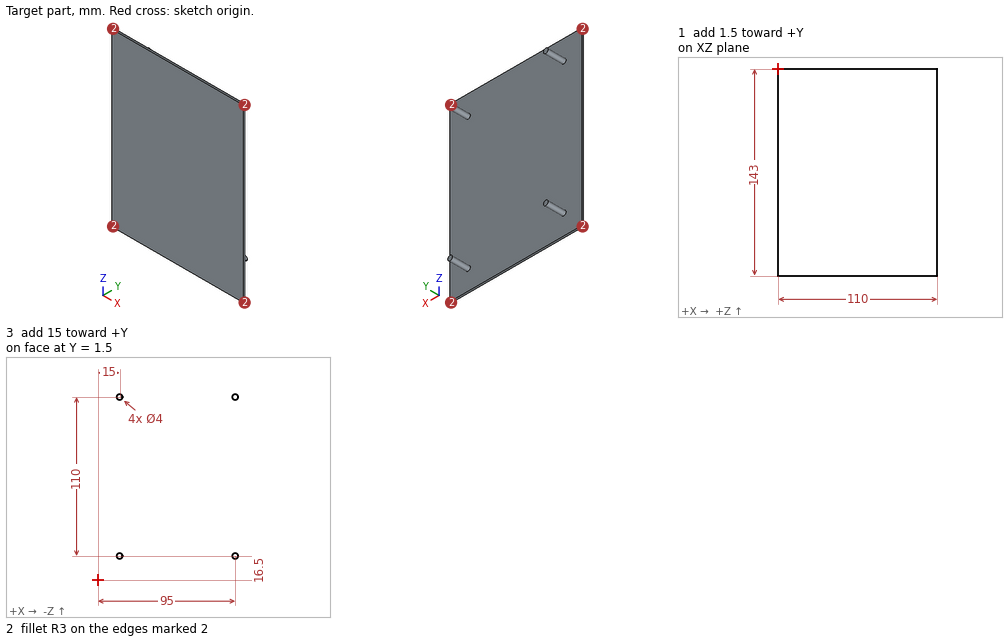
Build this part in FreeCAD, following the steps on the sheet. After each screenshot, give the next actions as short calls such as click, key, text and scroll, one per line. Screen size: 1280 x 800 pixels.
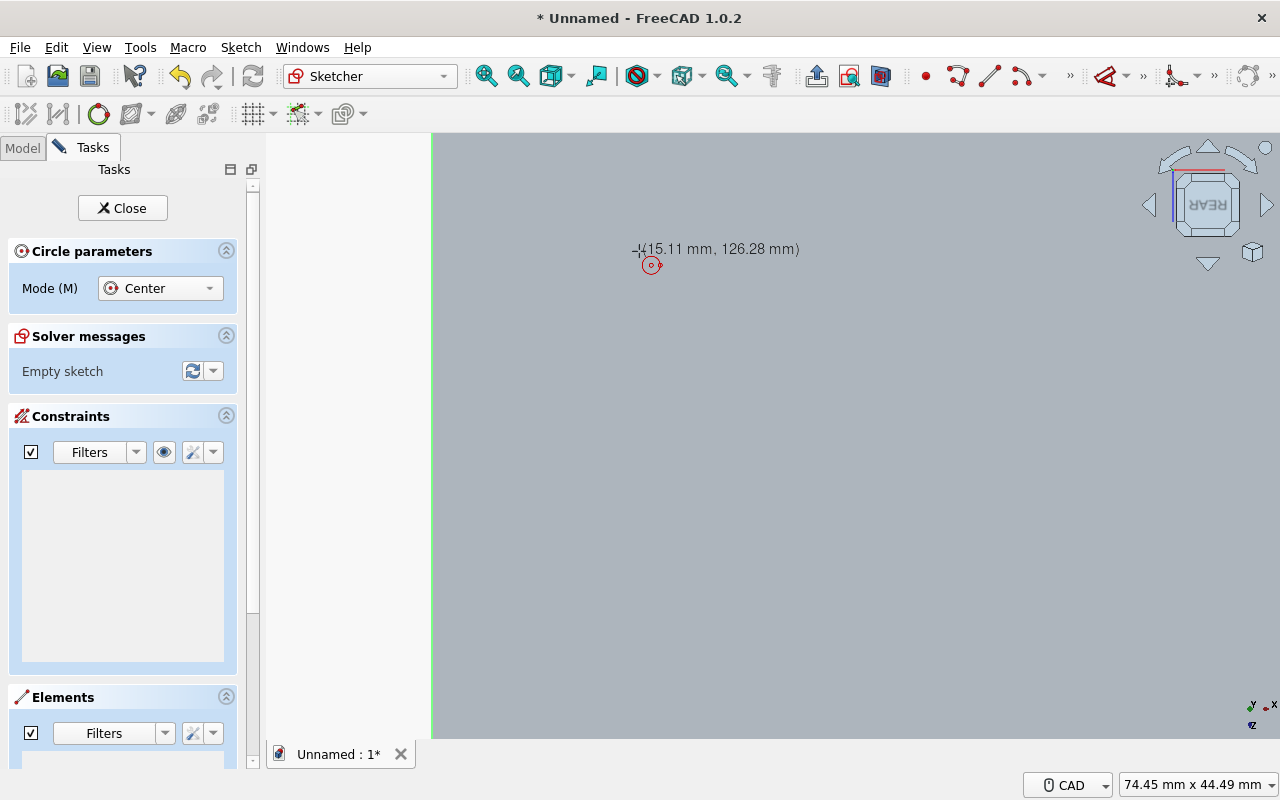
scroll(606, 268, down, 8)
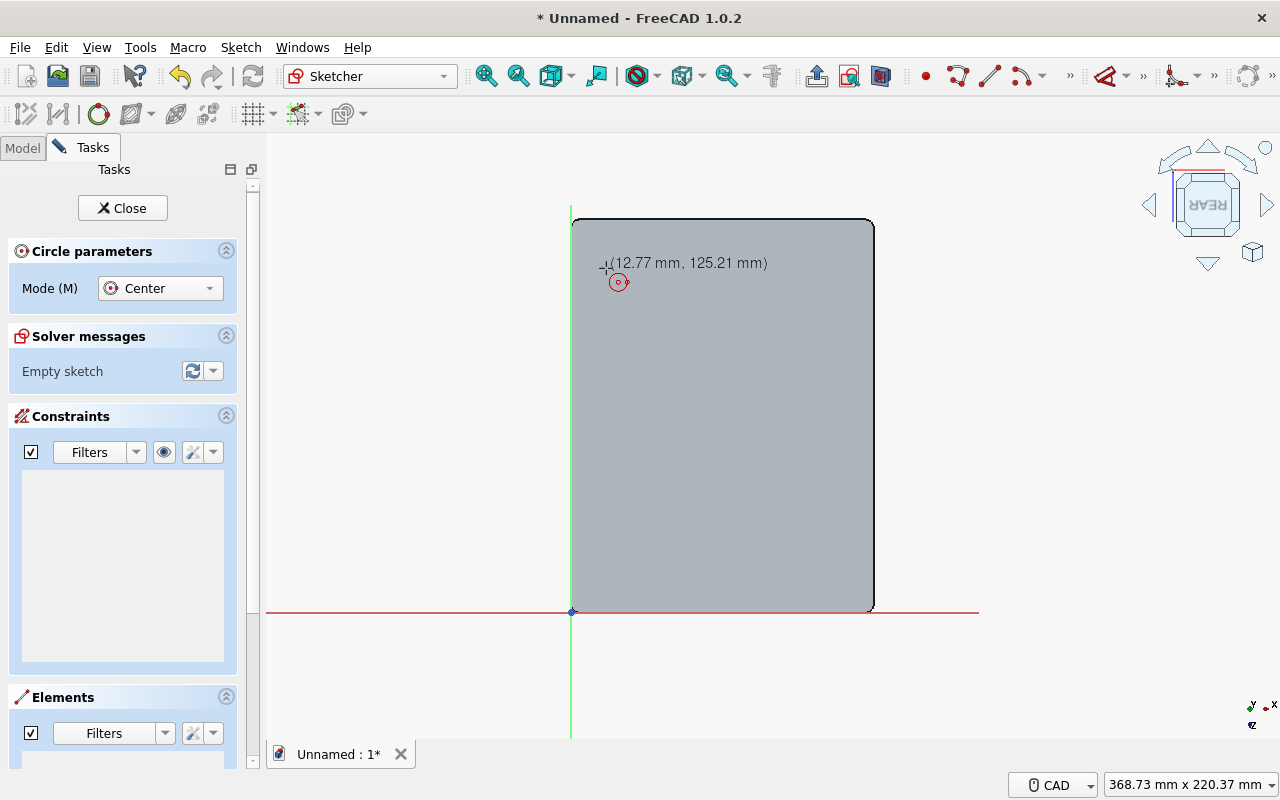
click(612, 265)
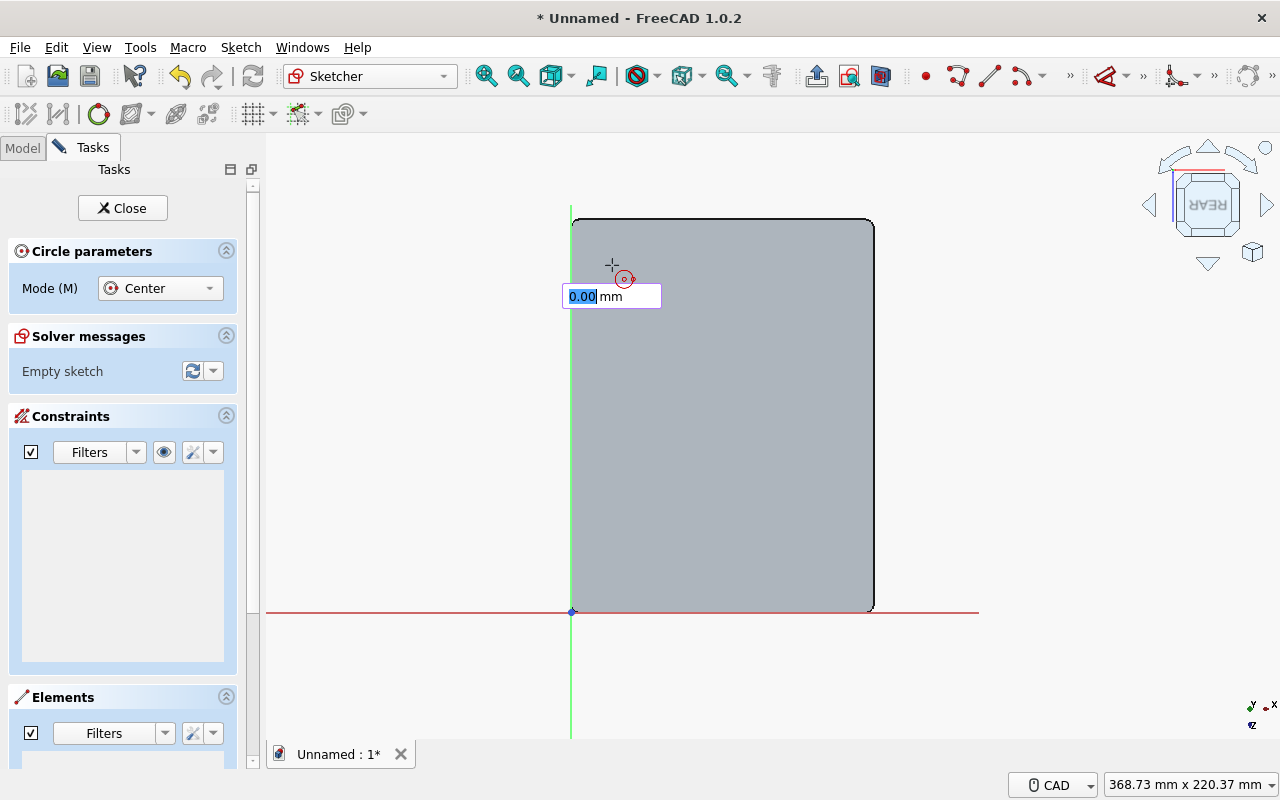
scroll(616, 261, up, 6)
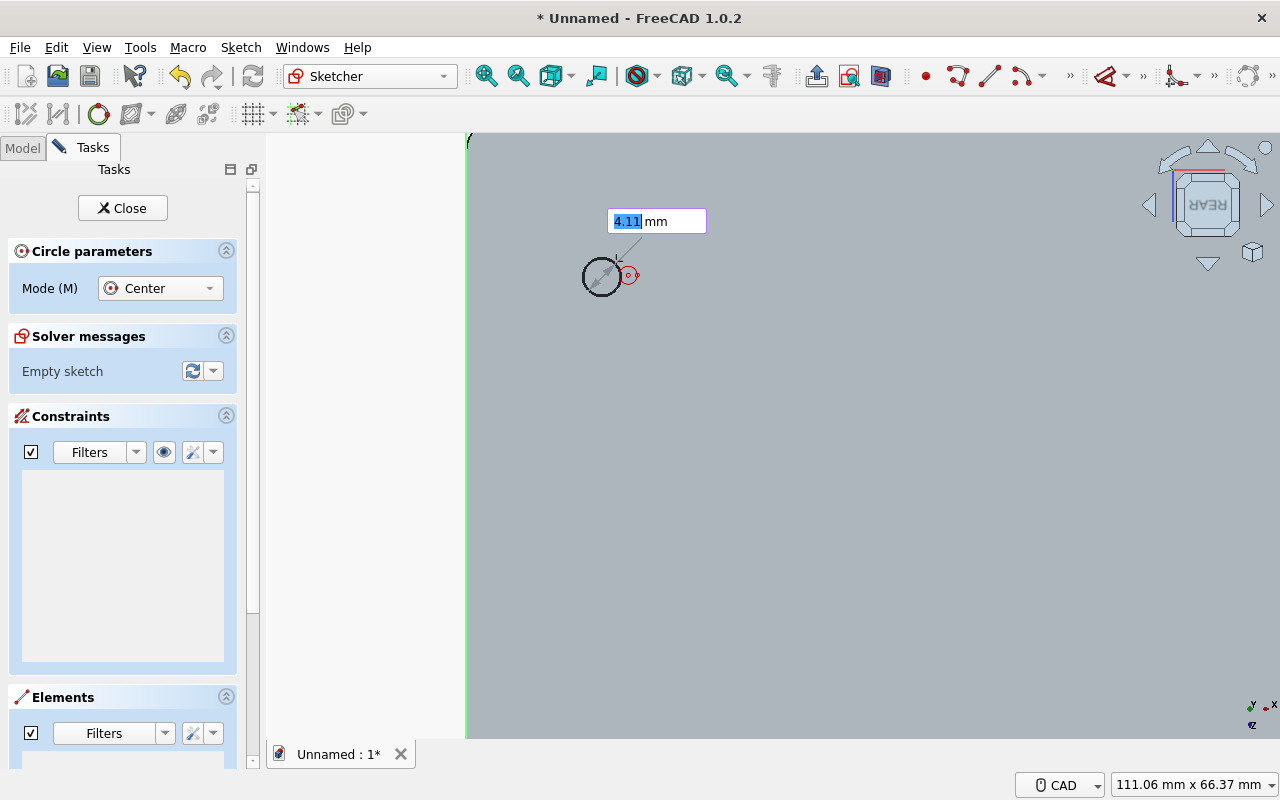
click(616, 260)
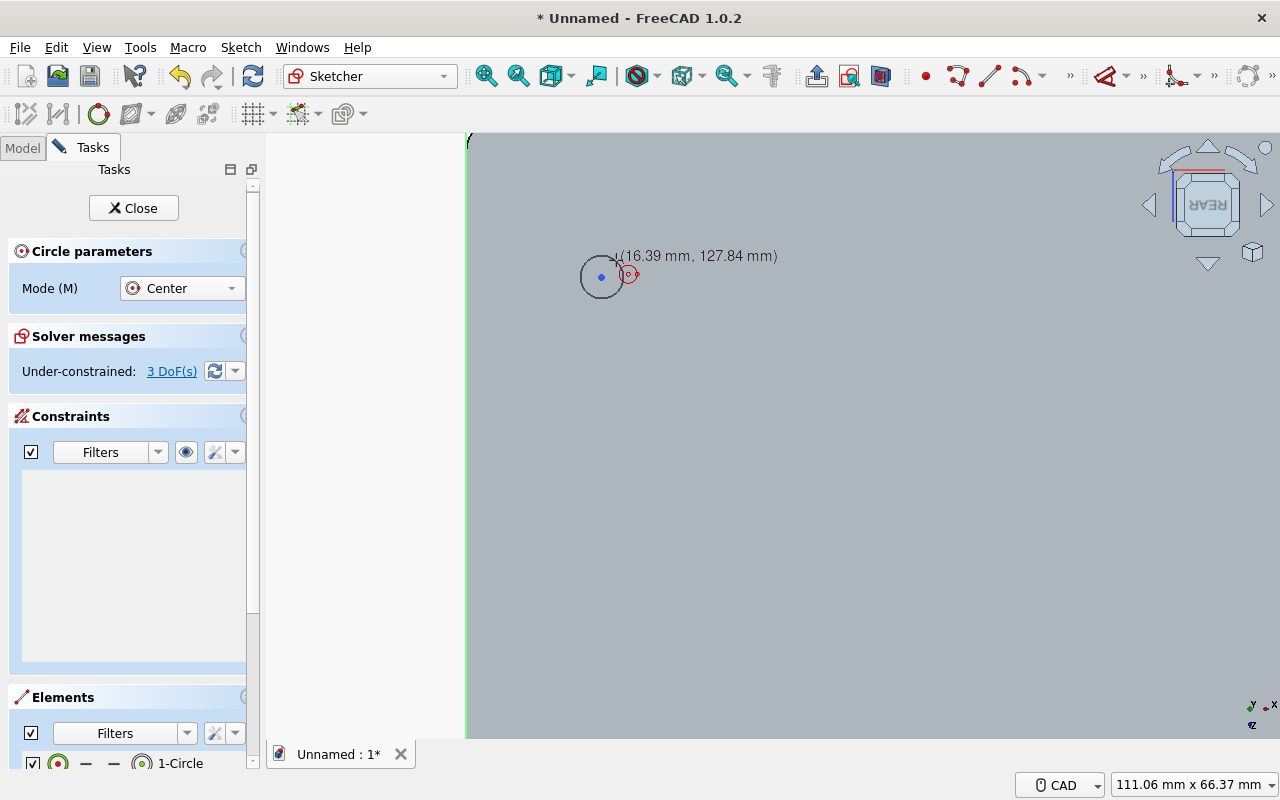
scroll(616, 261, down, 6)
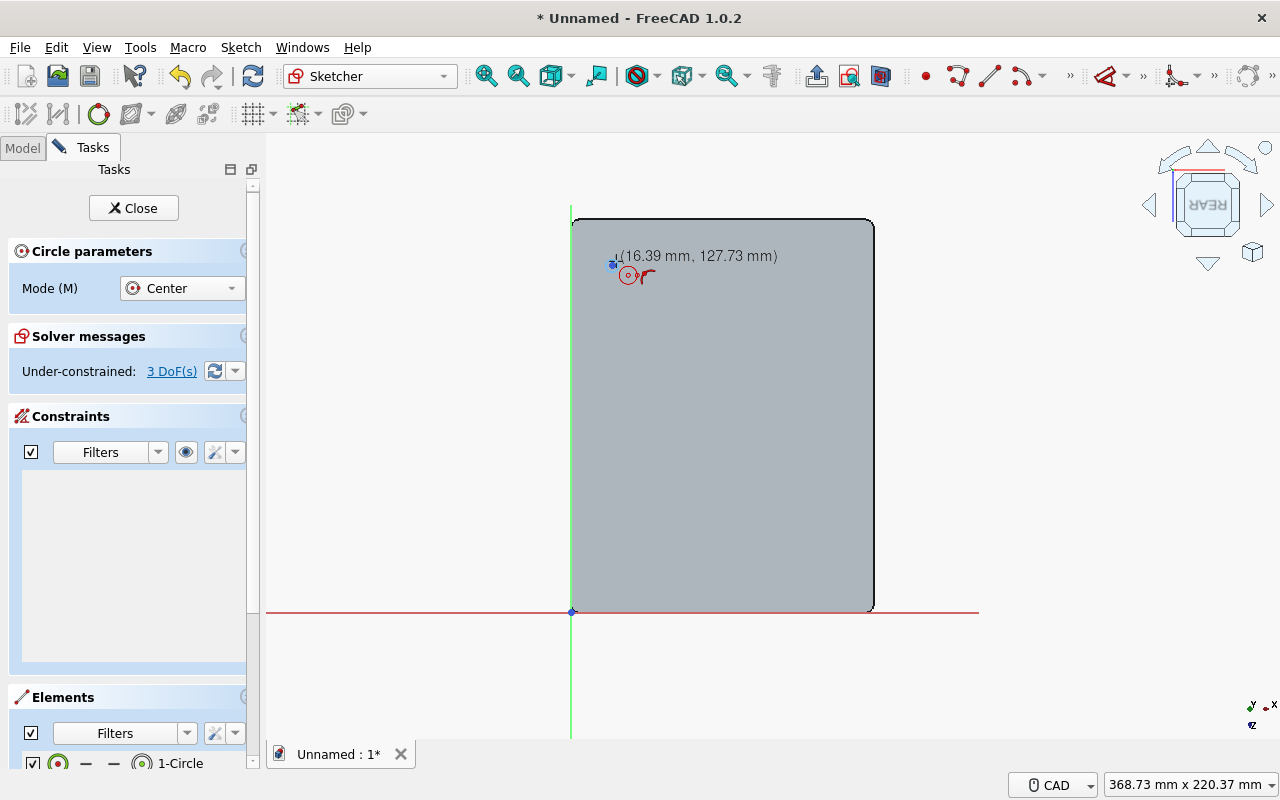
scroll(832, 567, up, 8)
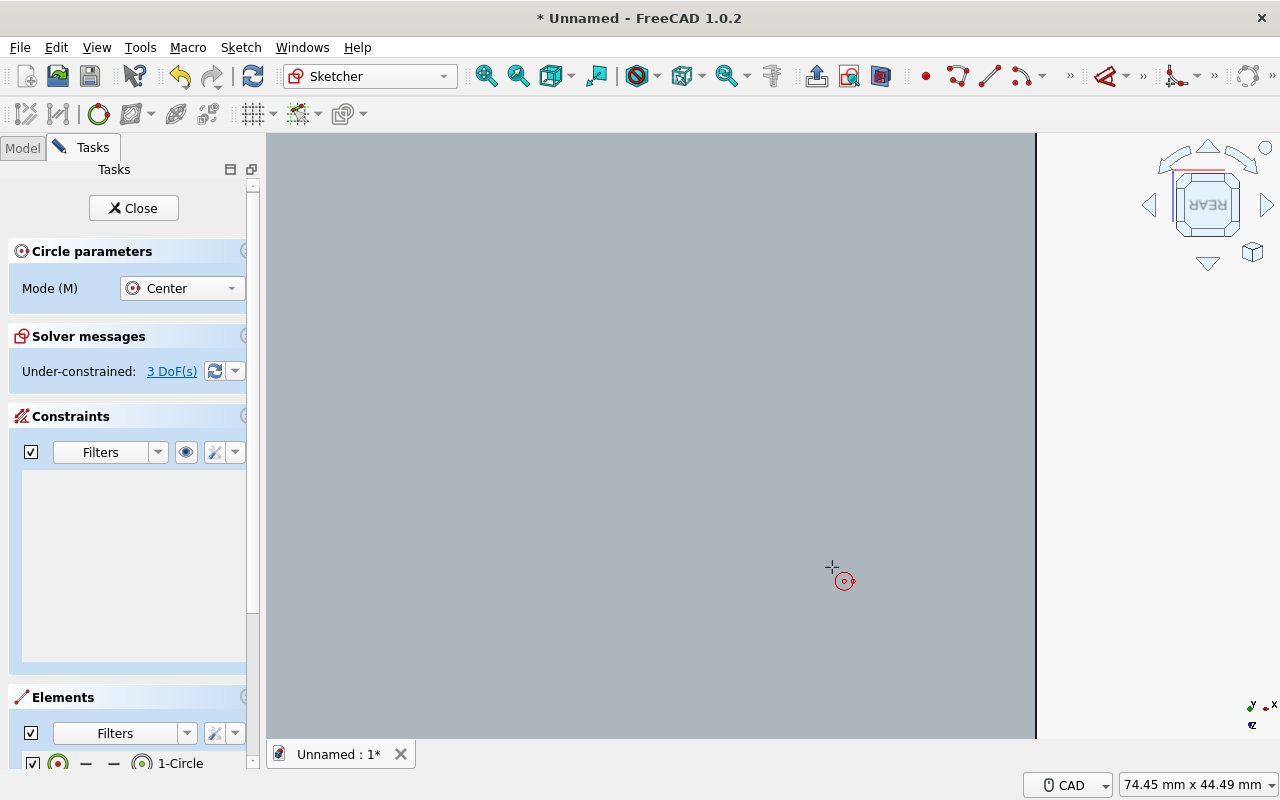
scroll(833, 568, down, 8)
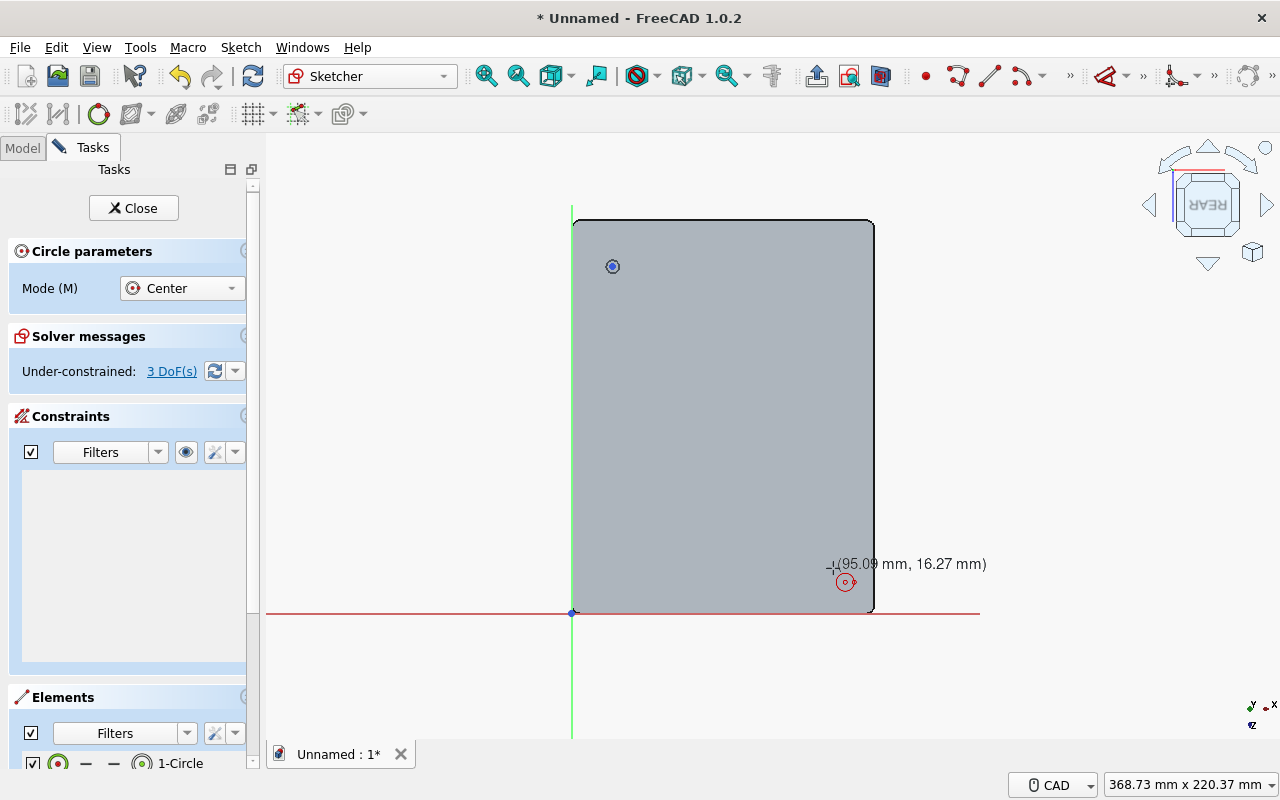
click(833, 568)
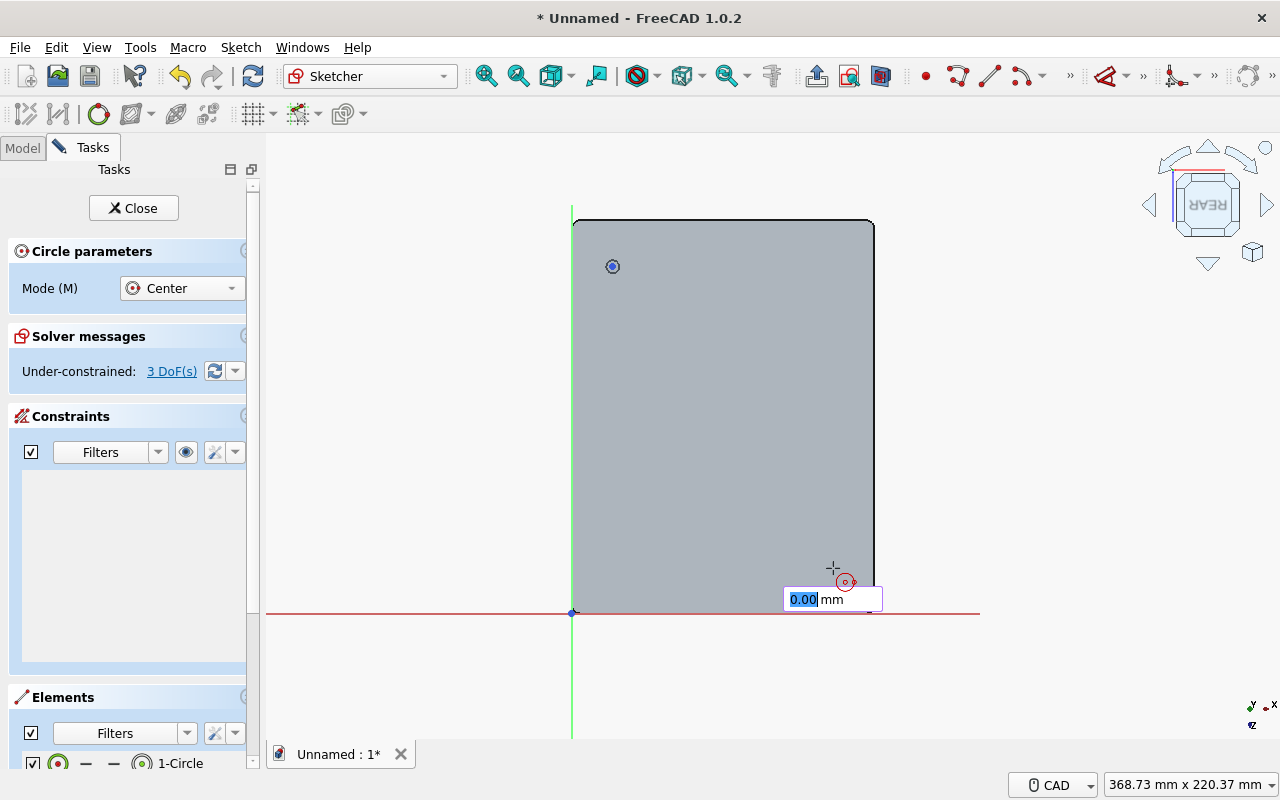
scroll(837, 564, up, 6)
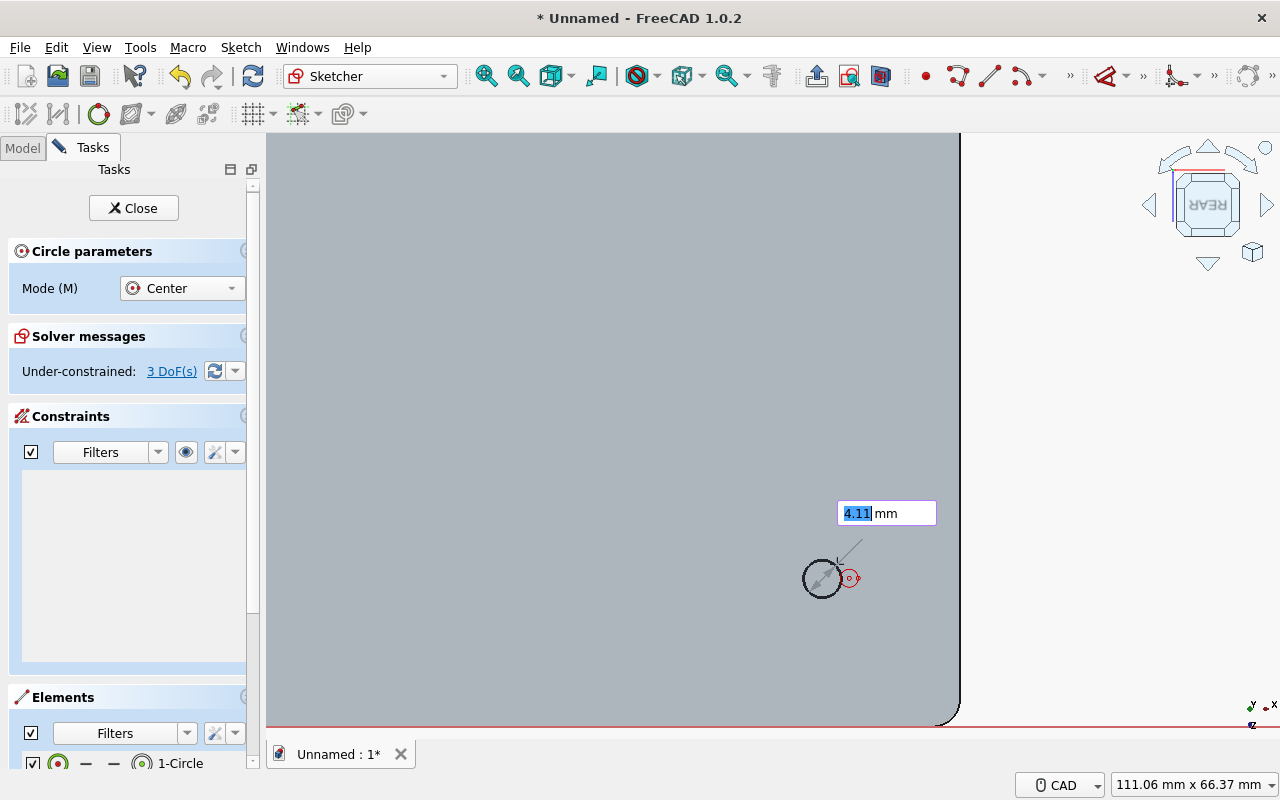
click(836, 563)